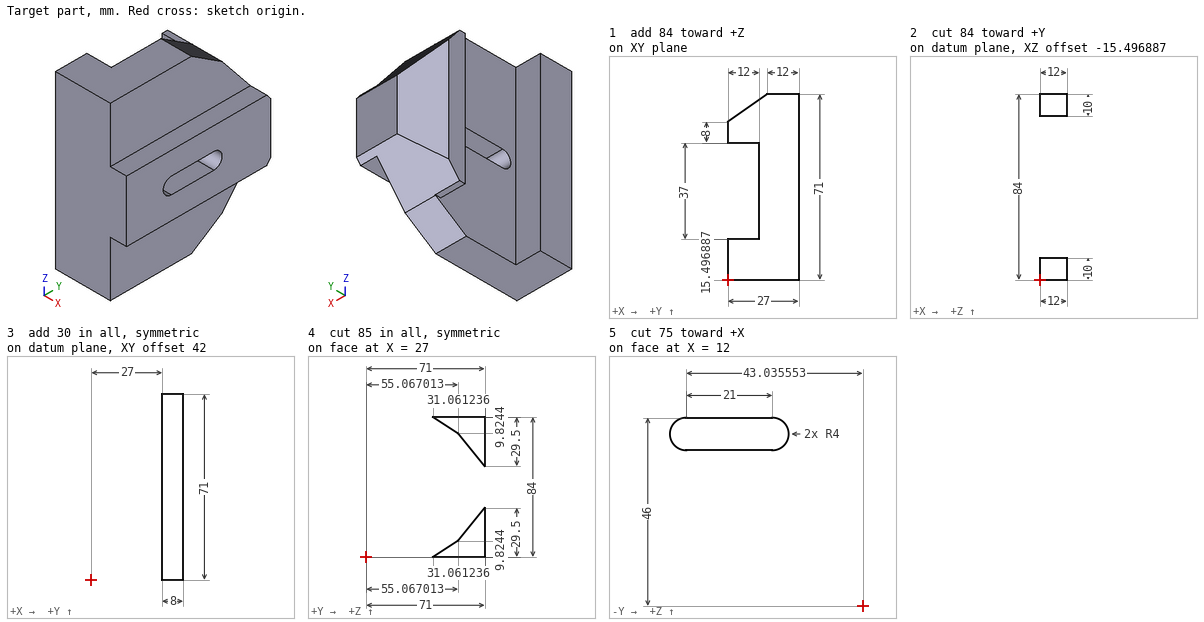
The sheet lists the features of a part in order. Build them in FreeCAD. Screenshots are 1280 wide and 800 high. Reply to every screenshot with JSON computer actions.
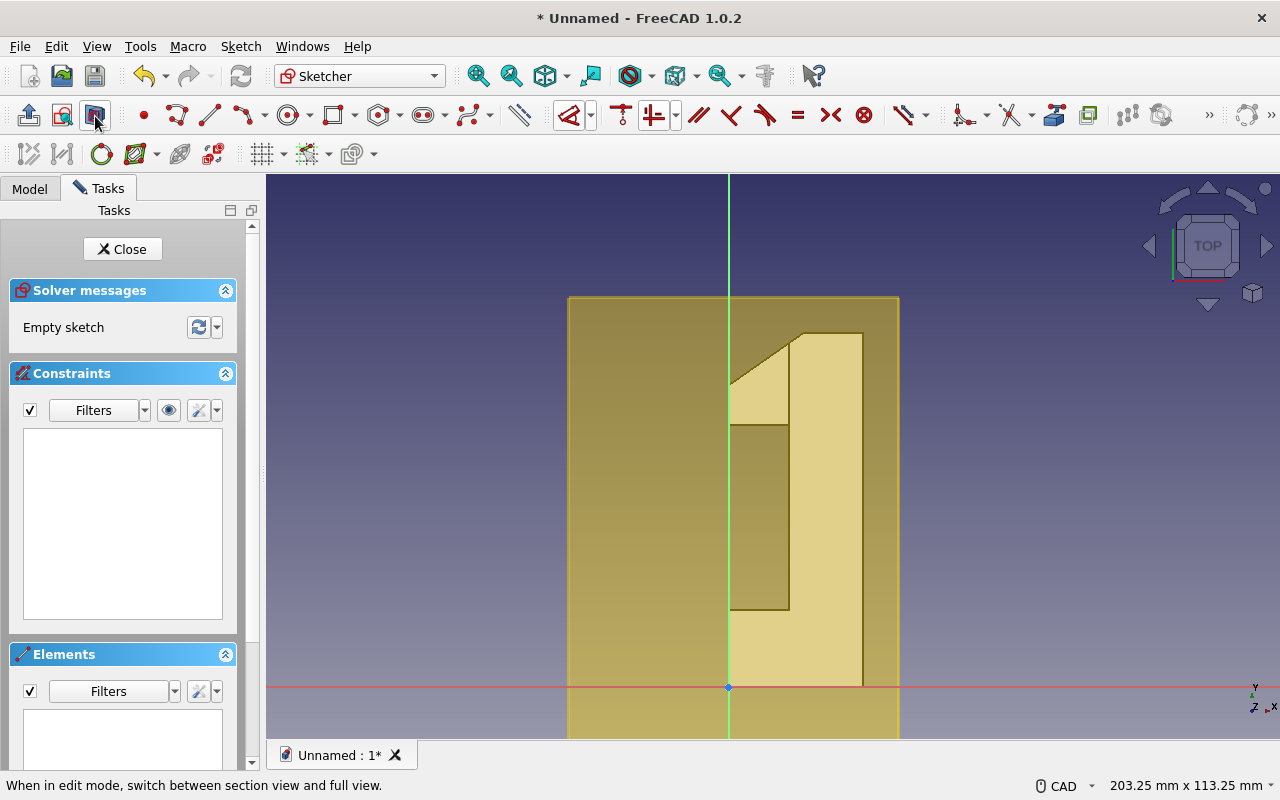
{"action": "scroll", "coordinate": [294, 214], "scroll_direction": "down", "scroll_amount": 1}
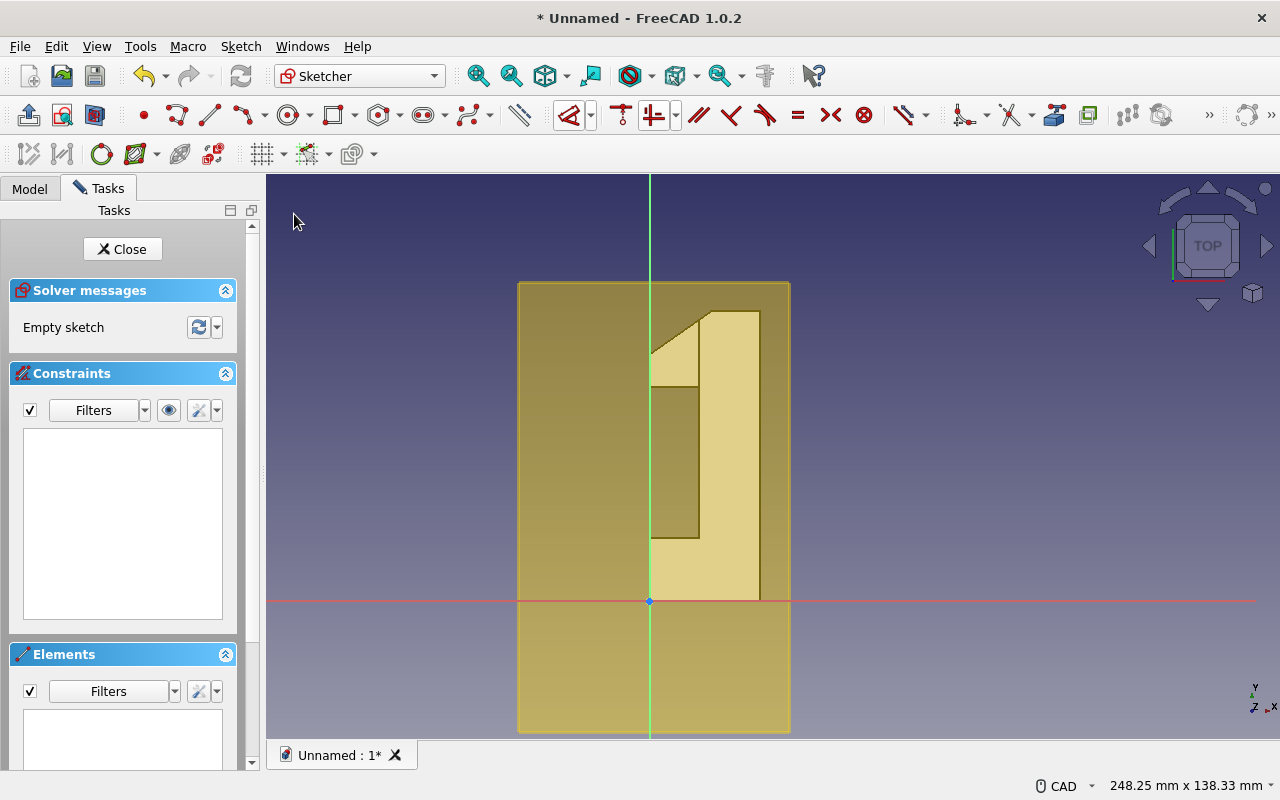
{"action": "left_click", "coordinate": [332, 116]}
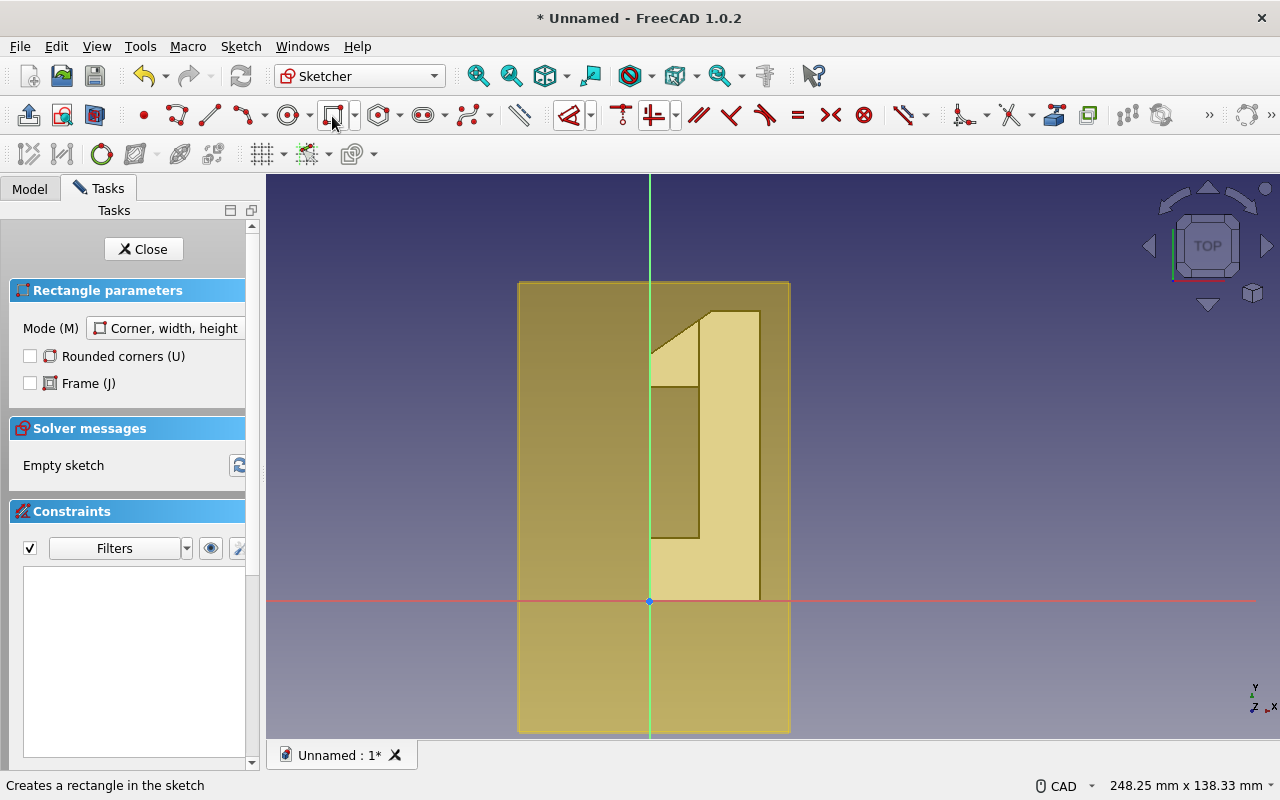
{"action": "left_click", "coordinate": [760, 311]}
{"action": "left_click", "coordinate": [793, 601]}
{"action": "key", "text": "Escape"}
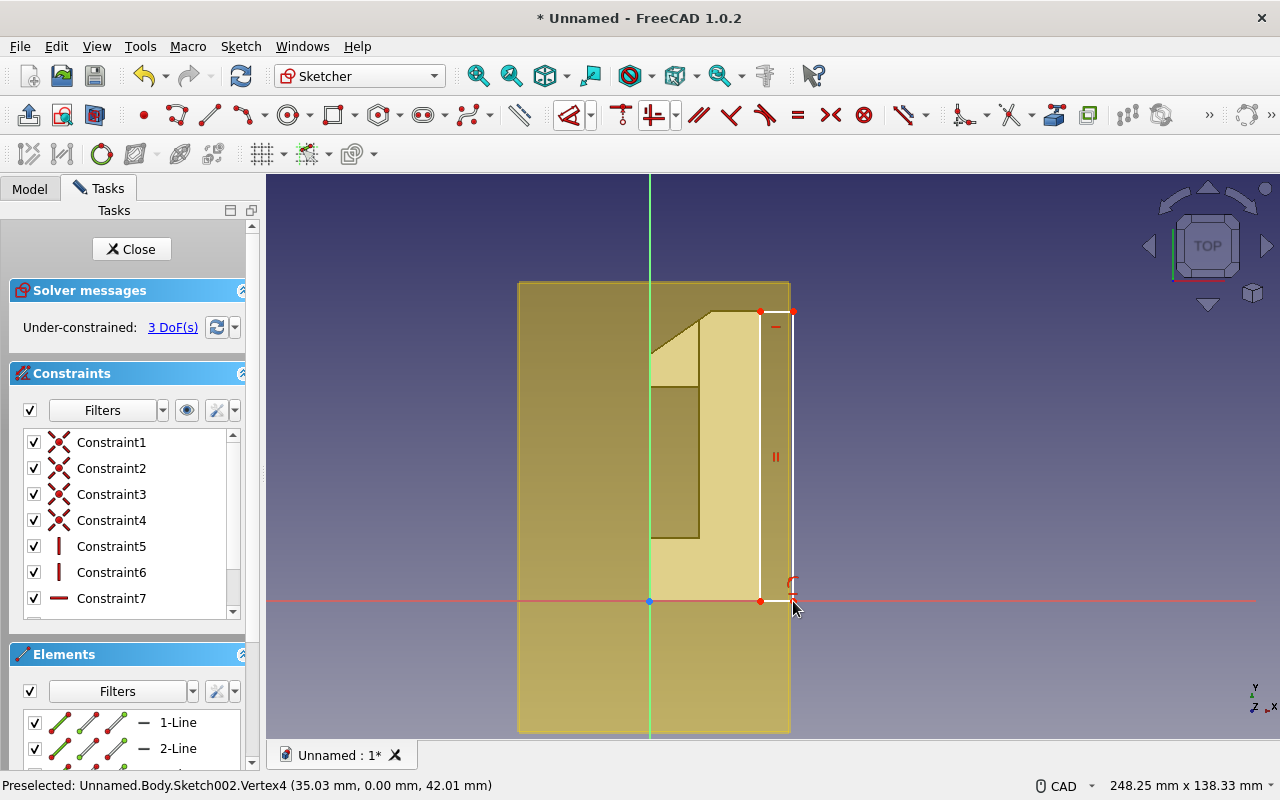
{"action": "scroll", "coordinate": [770, 601], "scroll_direction": "up", "scroll_amount": 2}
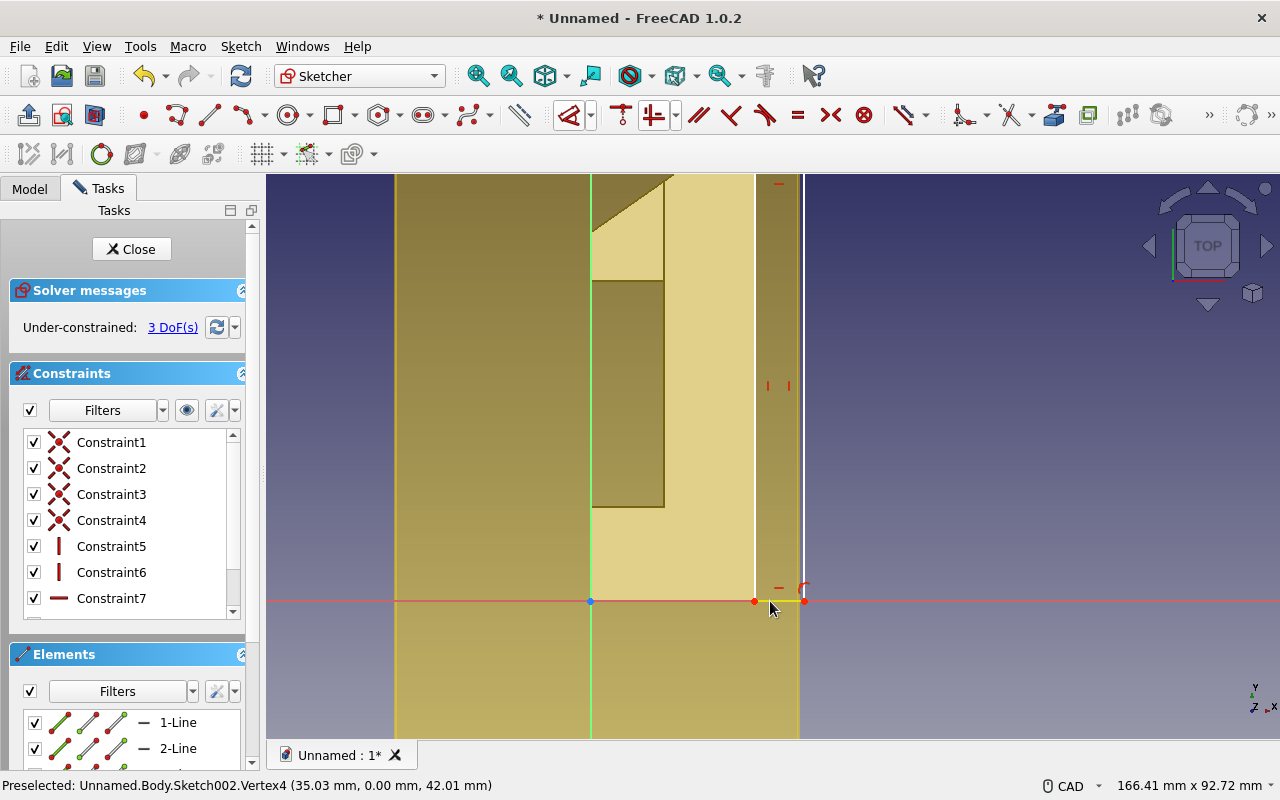
{"action": "left_click", "coordinate": [770, 601]}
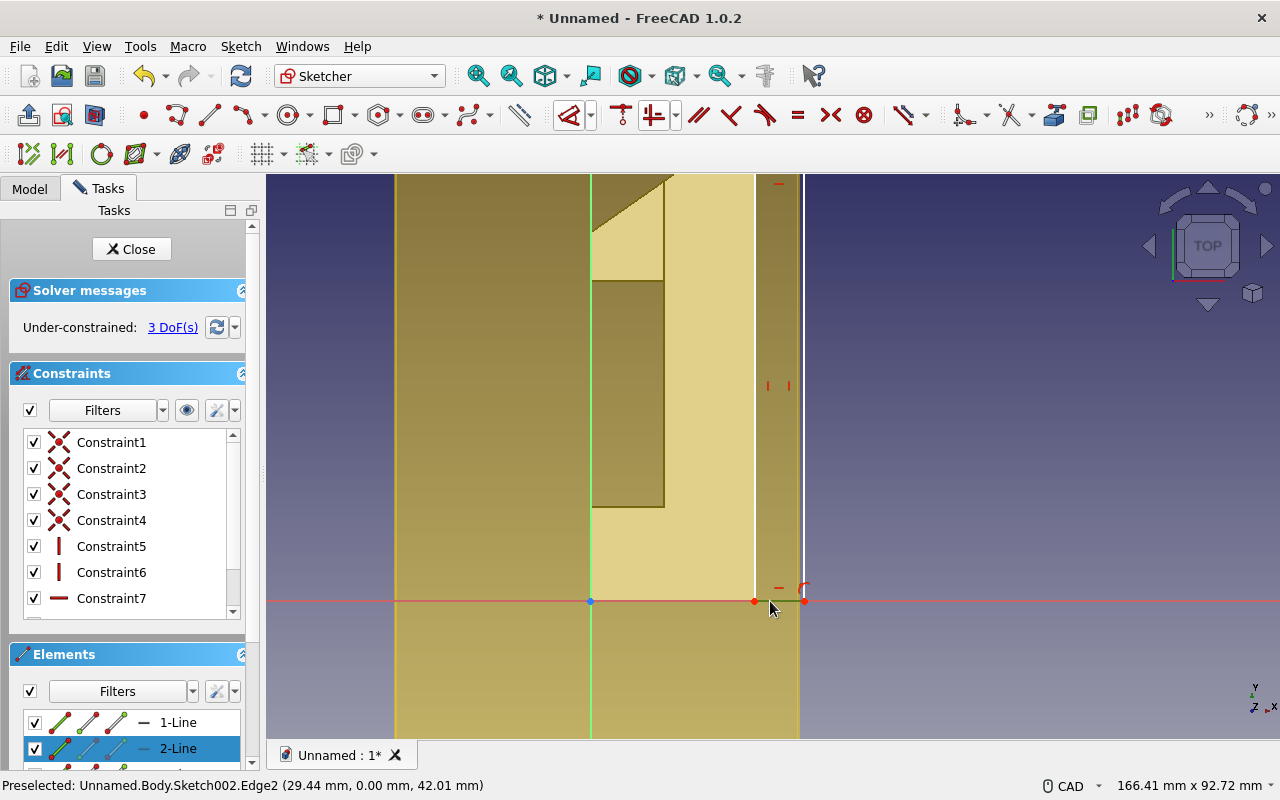
{"action": "left_click", "coordinate": [590, 116]}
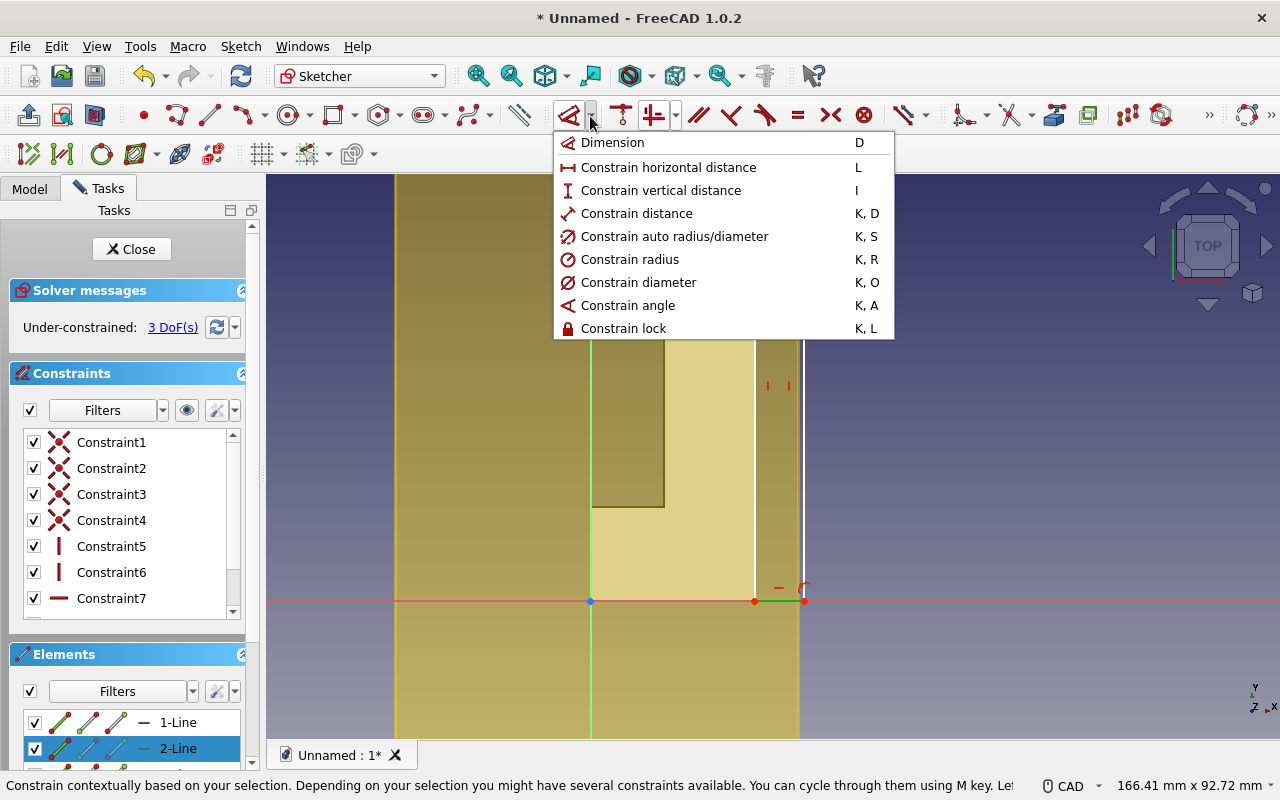
{"action": "left_click", "coordinate": [724, 168]}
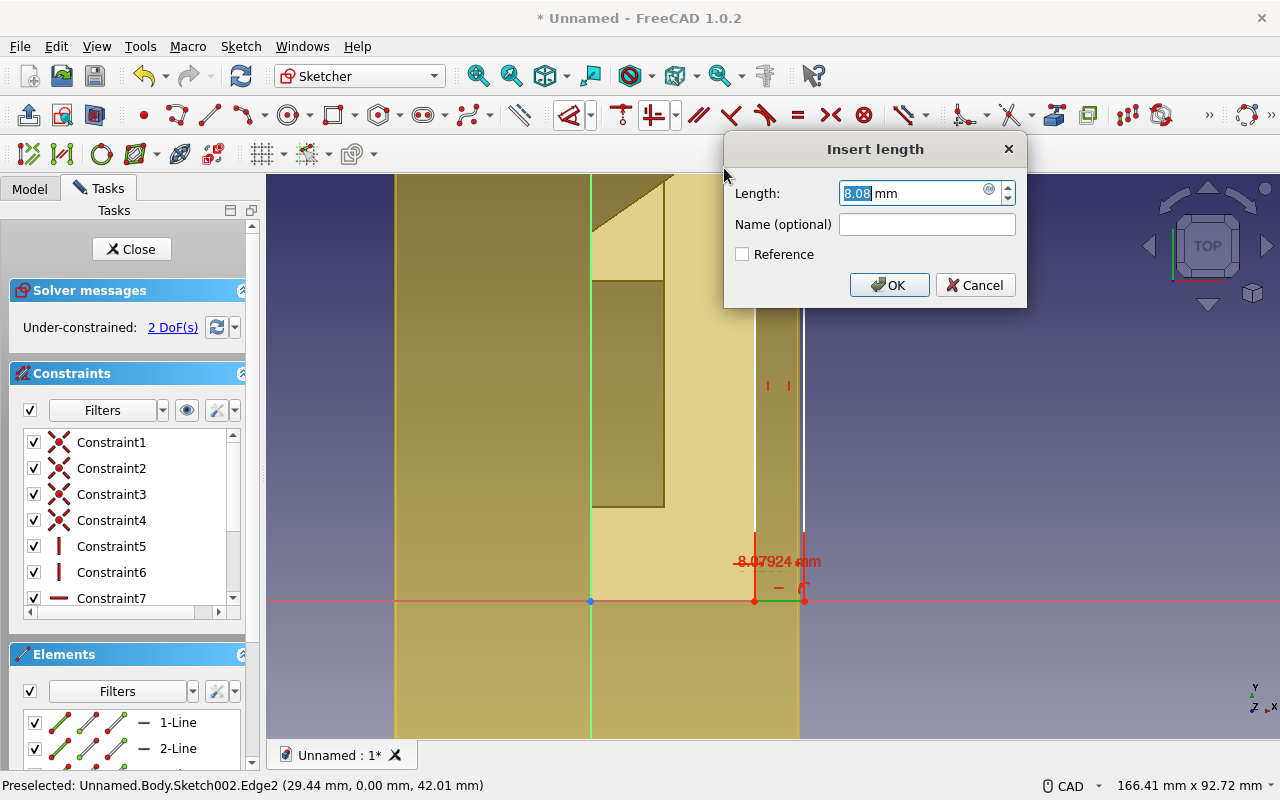
{"action": "type", "text": "8"}
{"action": "key", "text": "Return"}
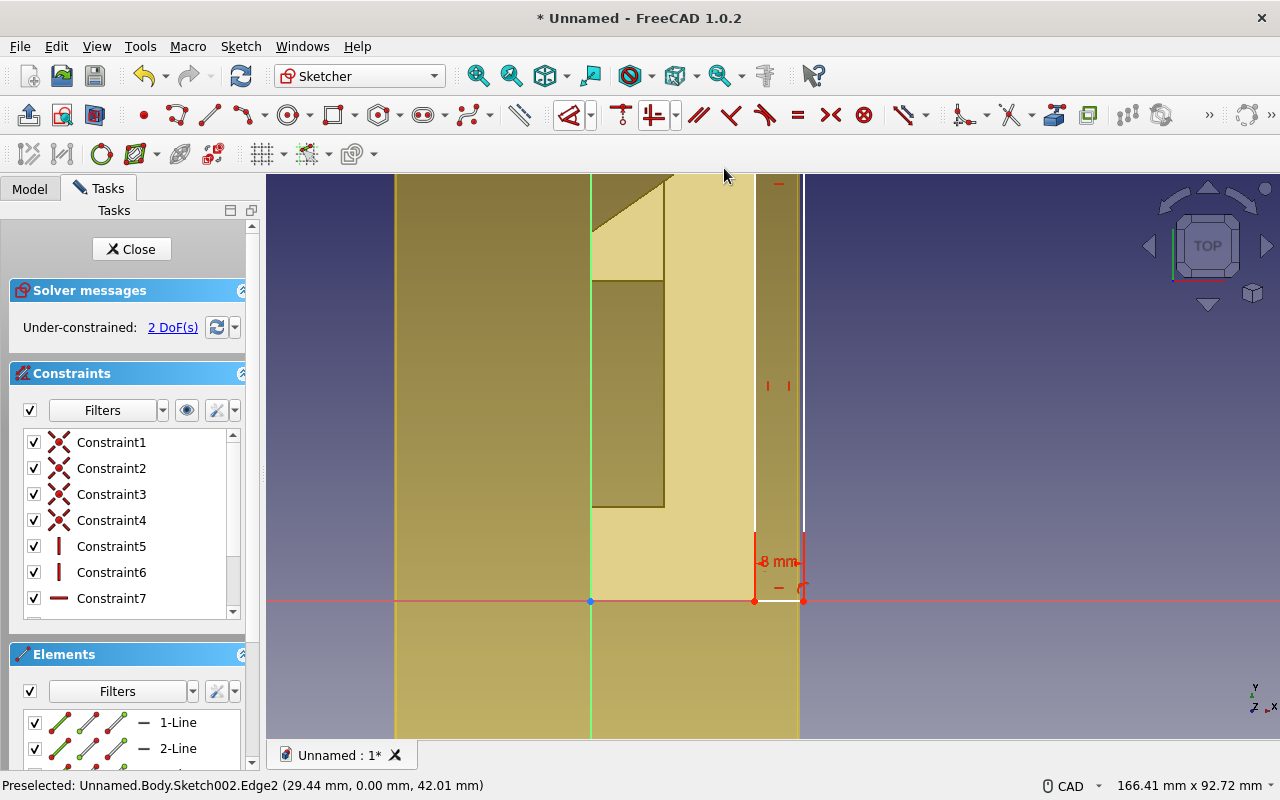
{"action": "left_click", "coordinate": [755, 299]}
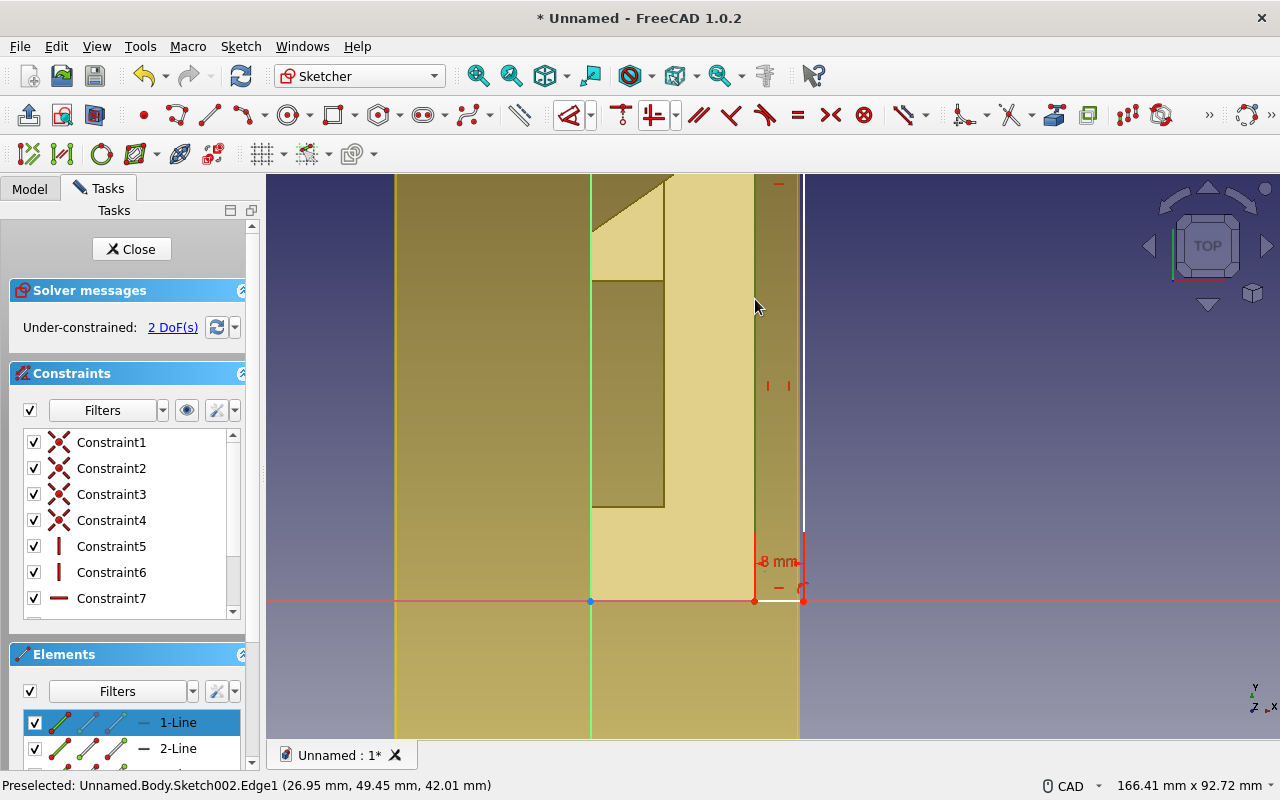
{"action": "left_click", "coordinate": [590, 116]}